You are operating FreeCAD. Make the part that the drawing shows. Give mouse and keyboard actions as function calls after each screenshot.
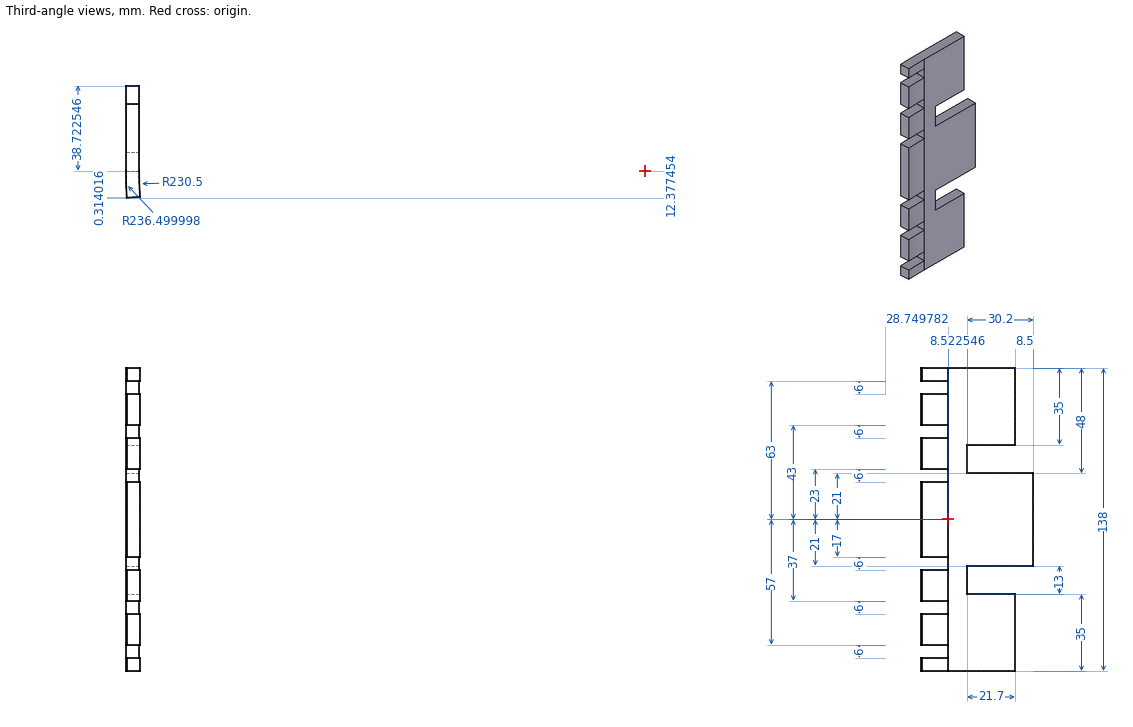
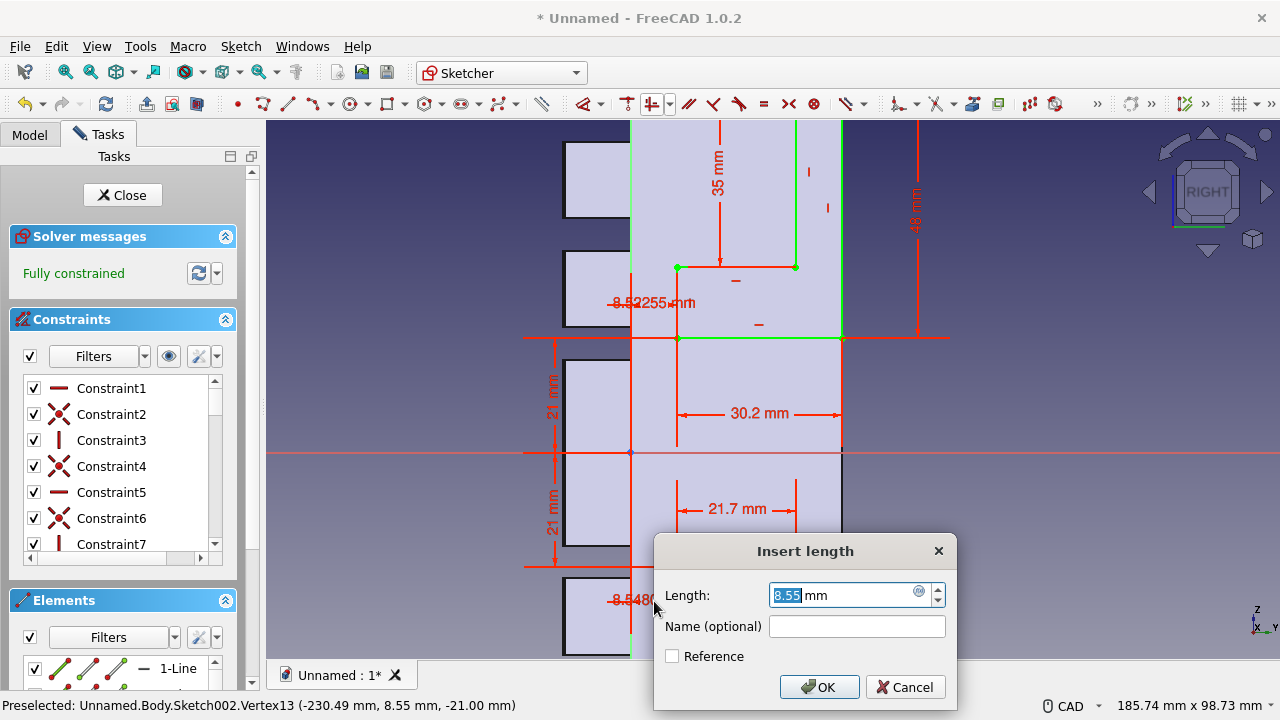
text(8.522546)
key(Return)
key(Escape)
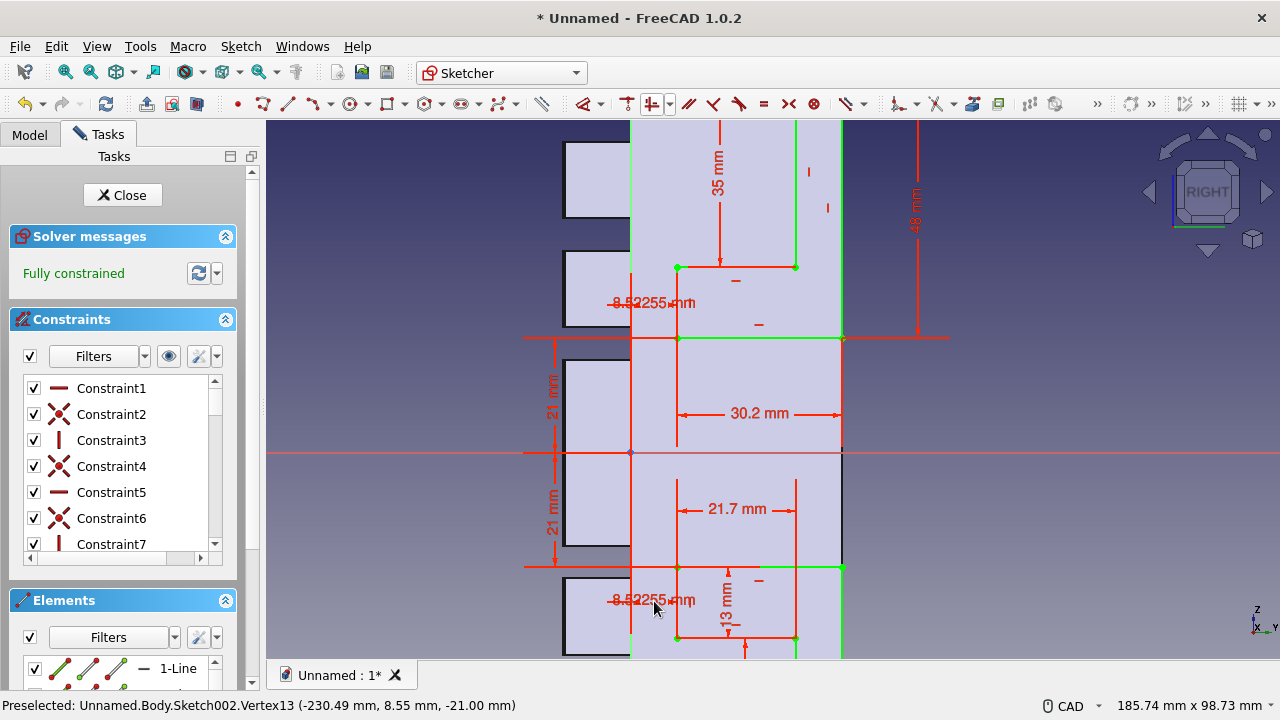
click(123, 195)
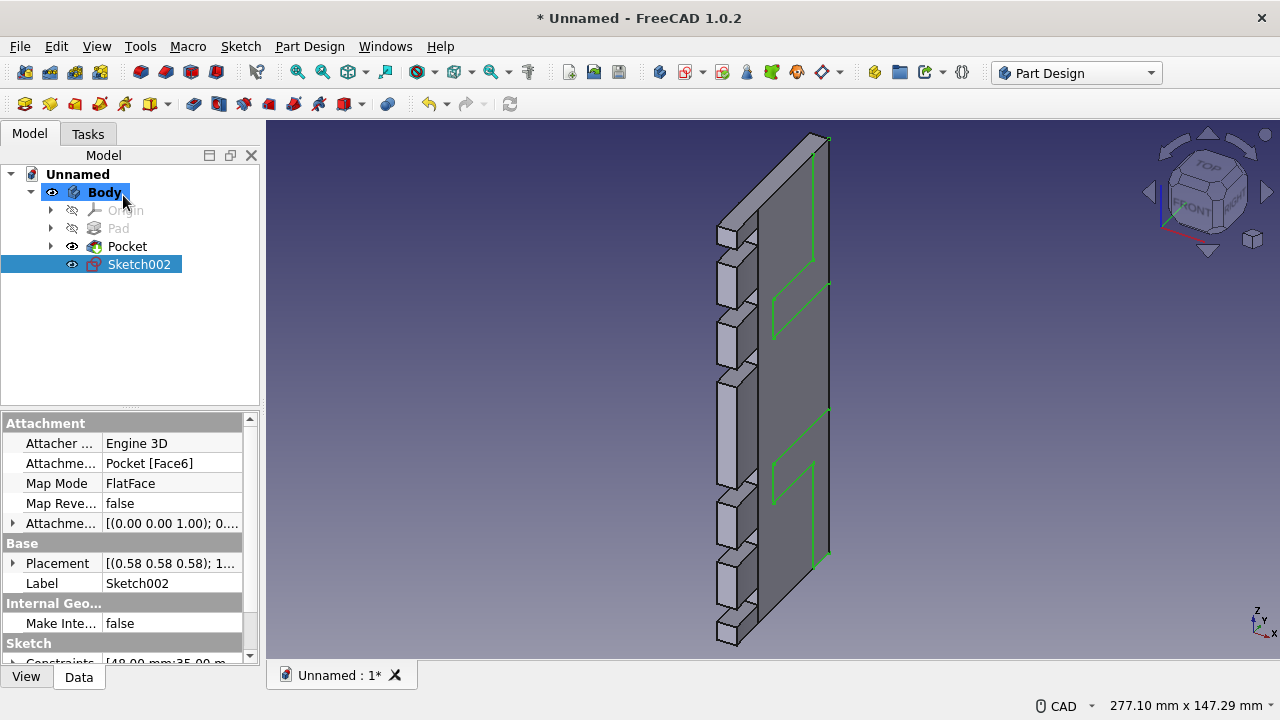
click(194, 104)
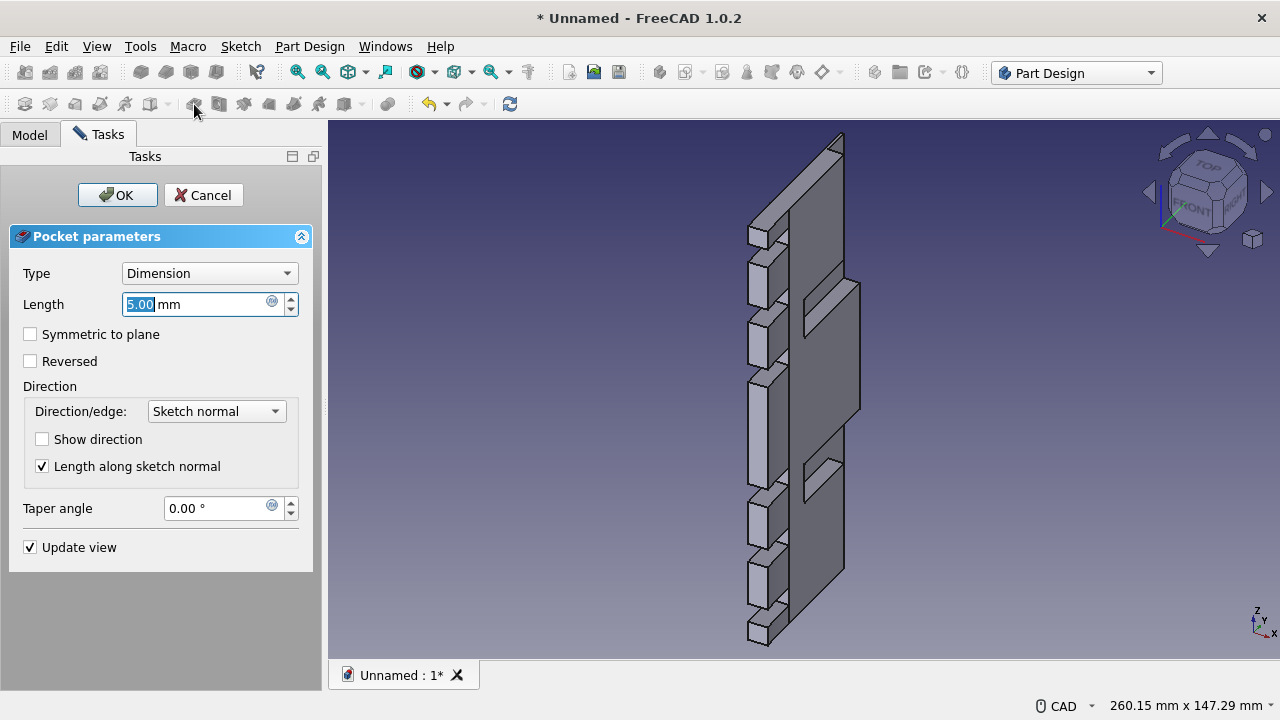
click(210, 274)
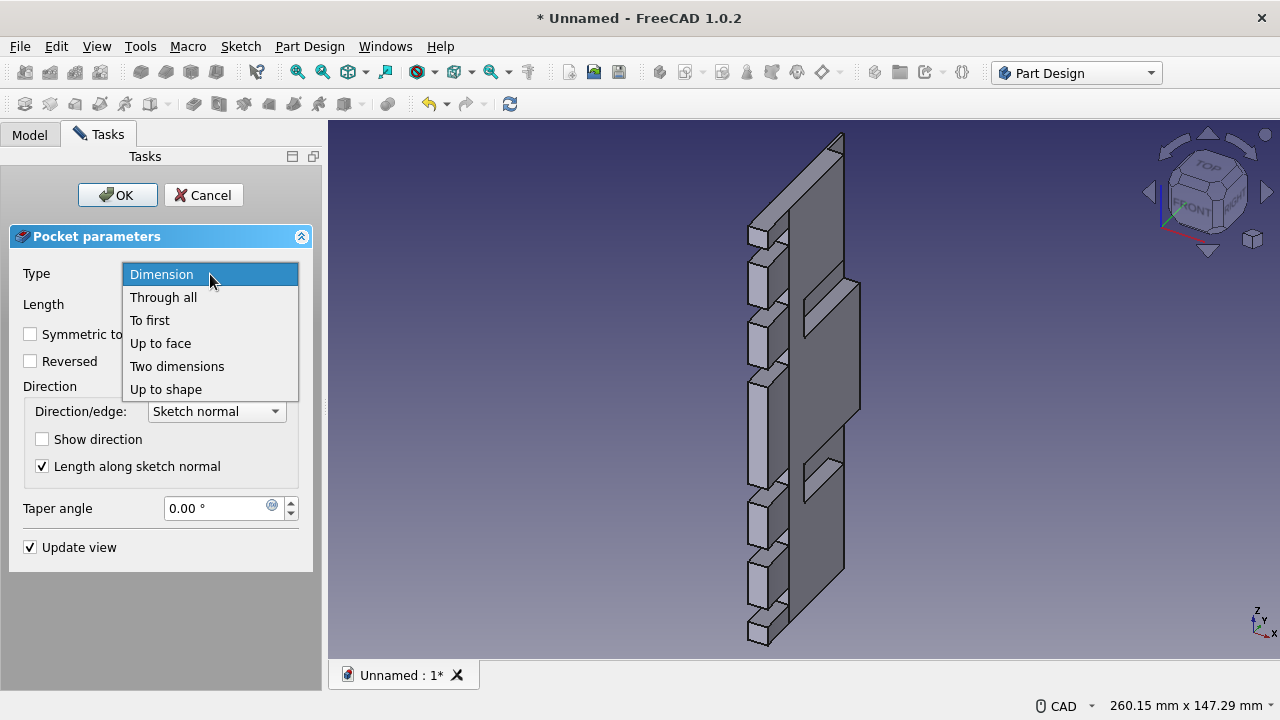
click(208, 298)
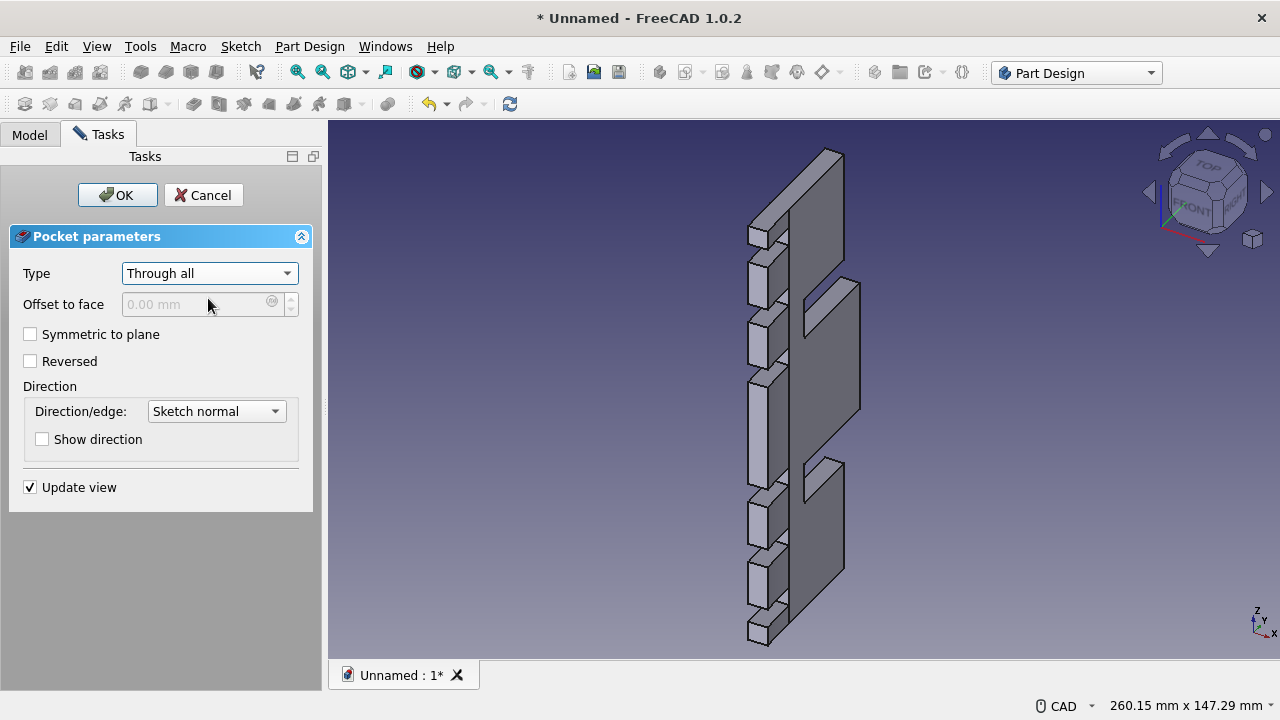
click(118, 195)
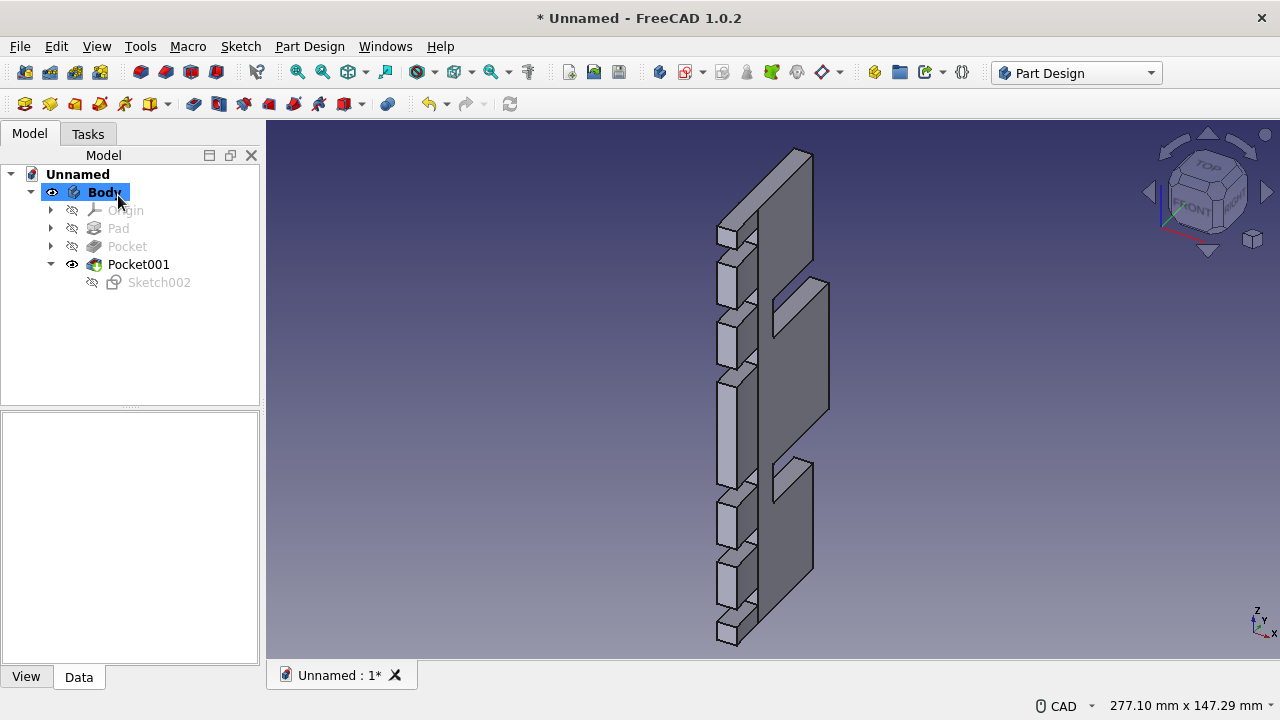
key(0)